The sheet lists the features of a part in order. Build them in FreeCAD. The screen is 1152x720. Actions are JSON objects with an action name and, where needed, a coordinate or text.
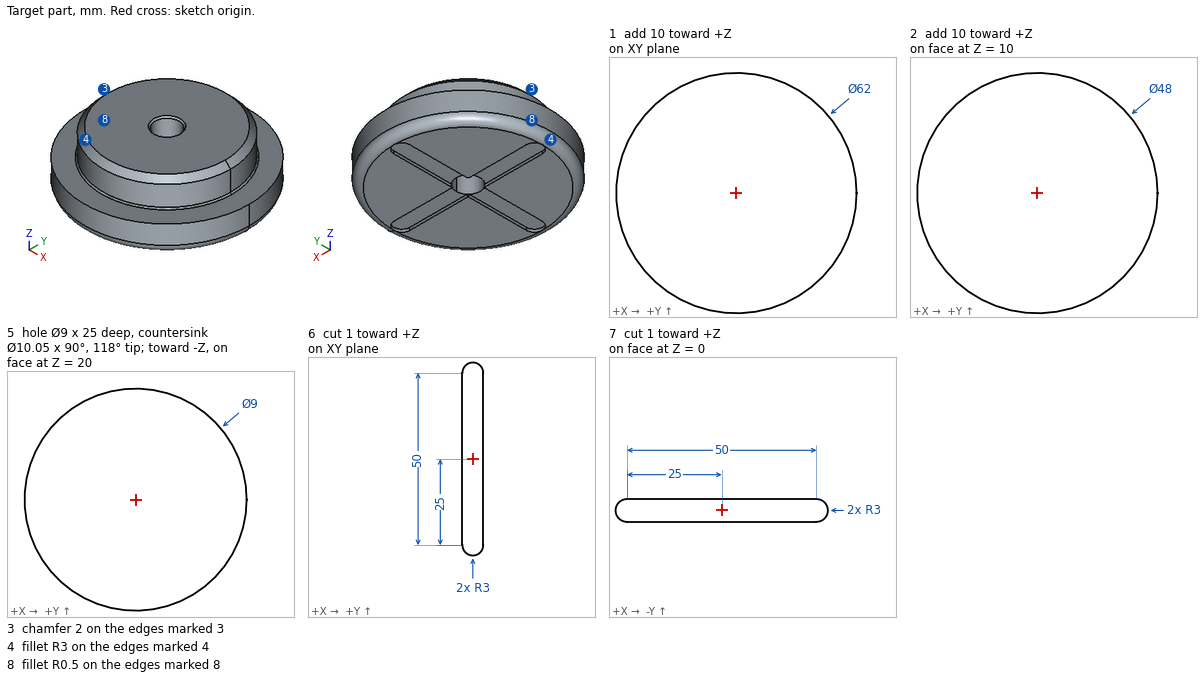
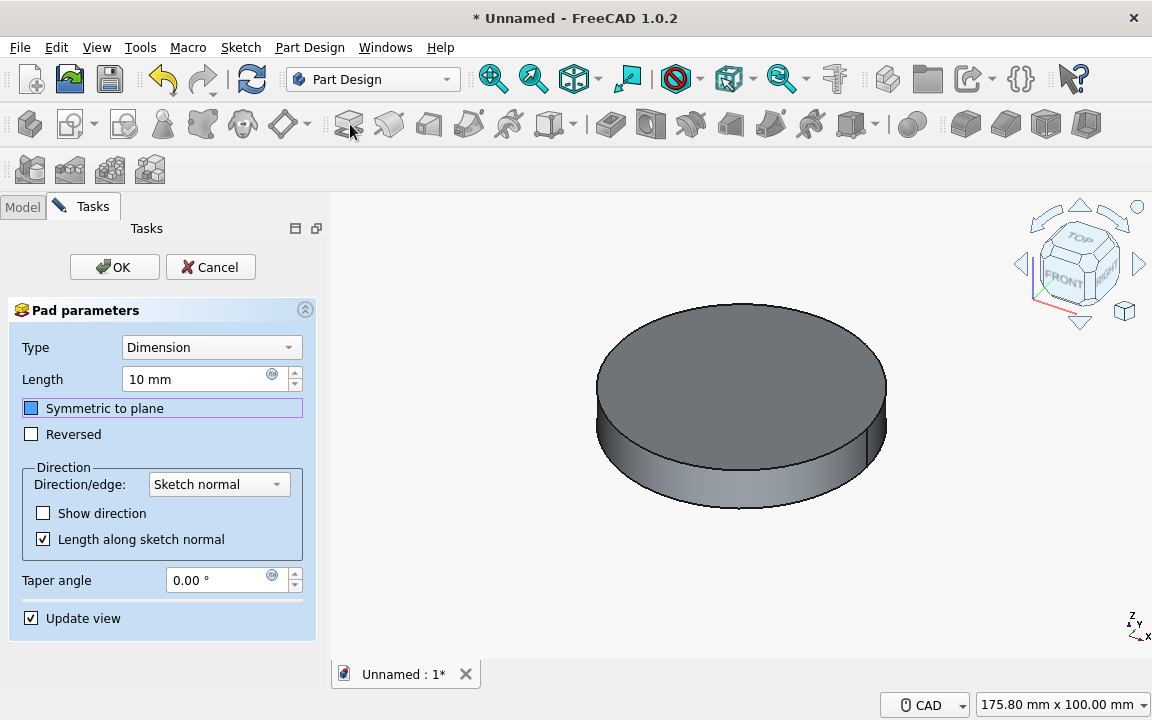
{"action": "left_click", "coordinate": [115, 267]}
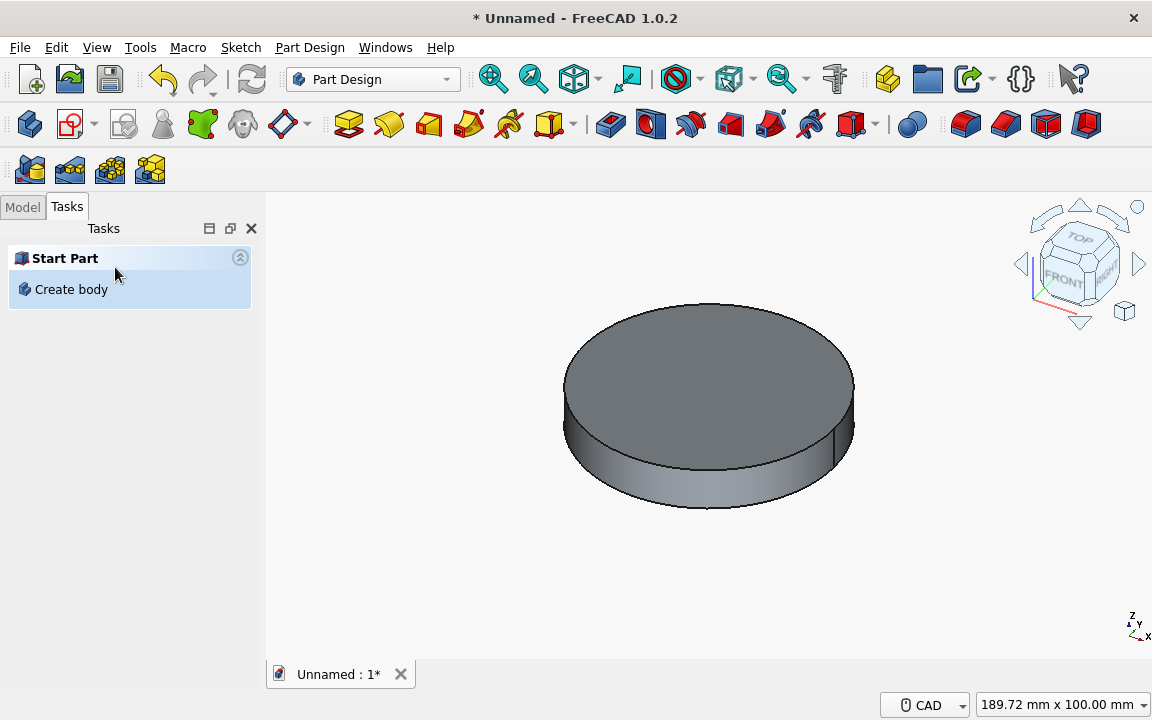
{"action": "left_click", "coordinate": [709, 386]}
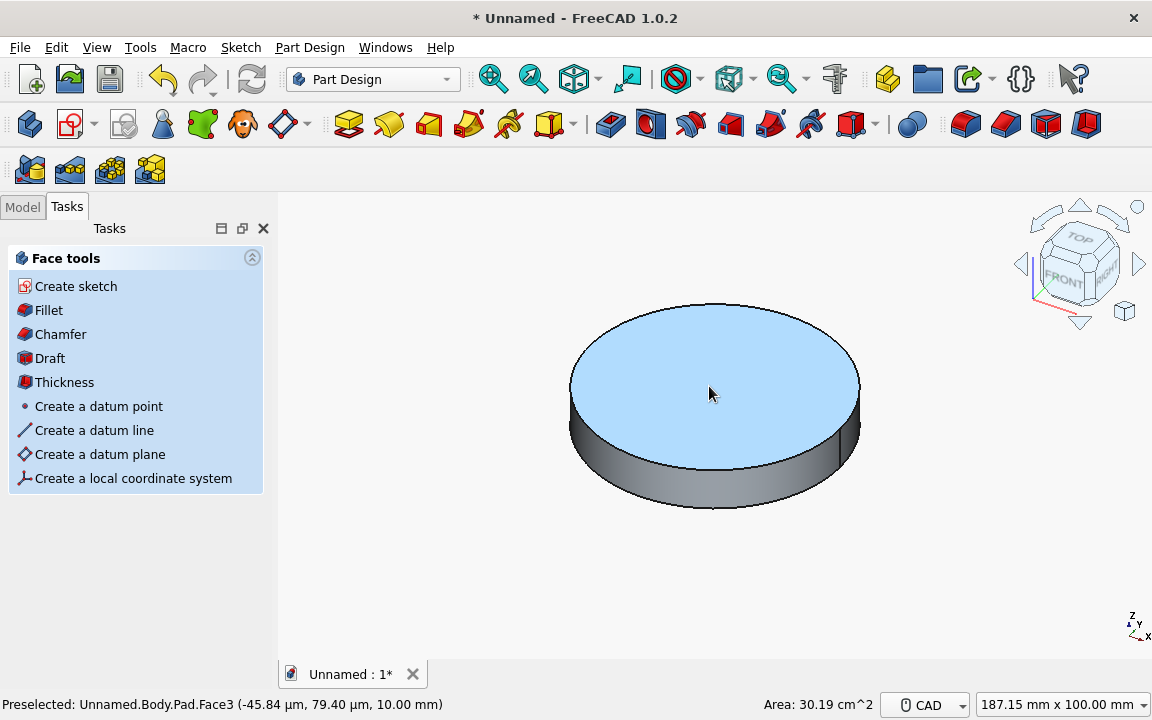
{"action": "left_click", "coordinate": [70, 124]}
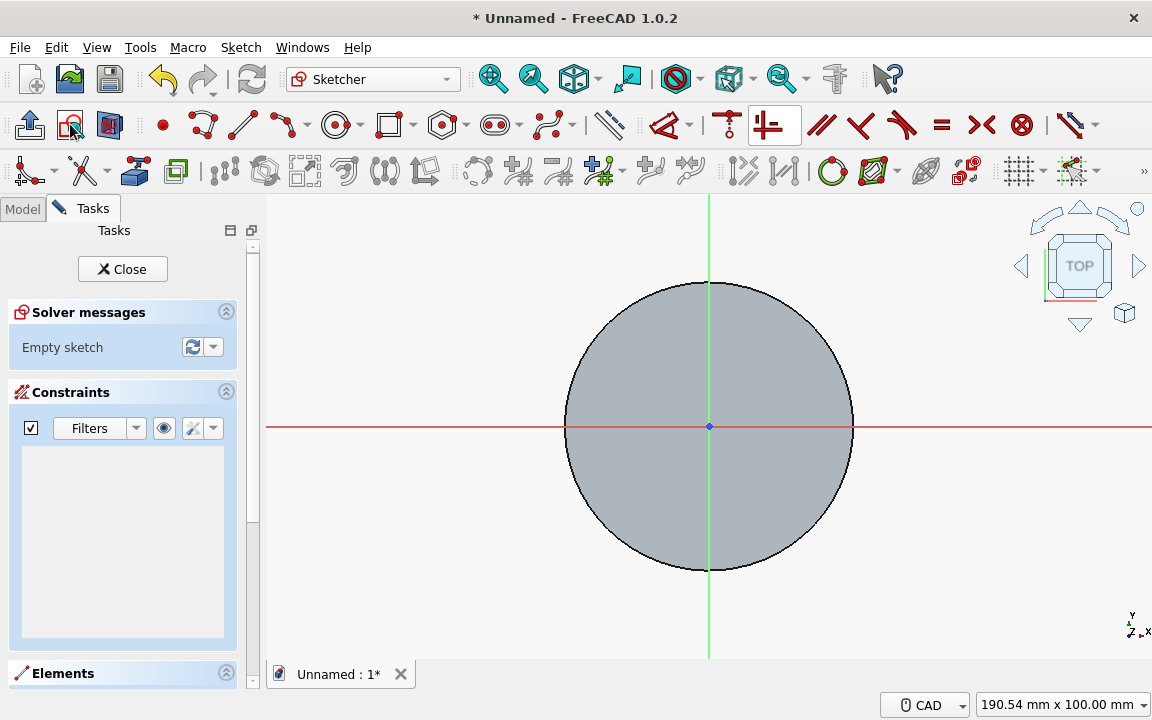
{"action": "key", "text": "g c"}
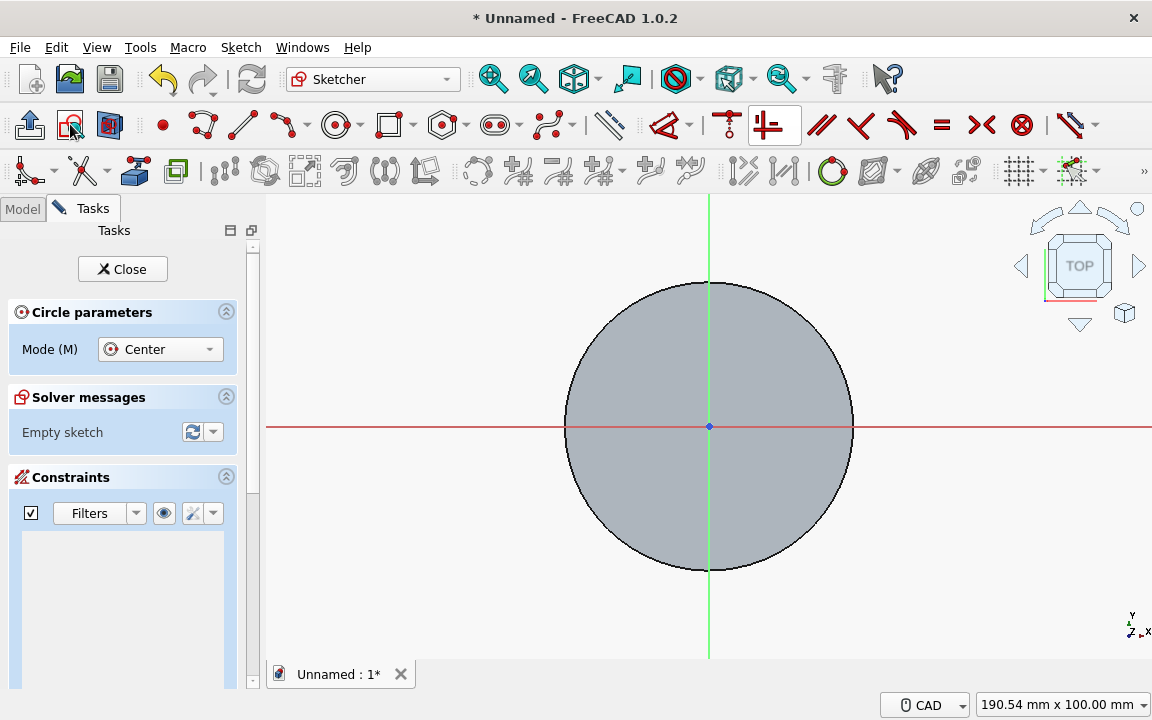
{"action": "left_click", "coordinate": [709, 426]}
{"action": "left_click", "coordinate": [788, 348]}
{"action": "key", "text": "Escape"}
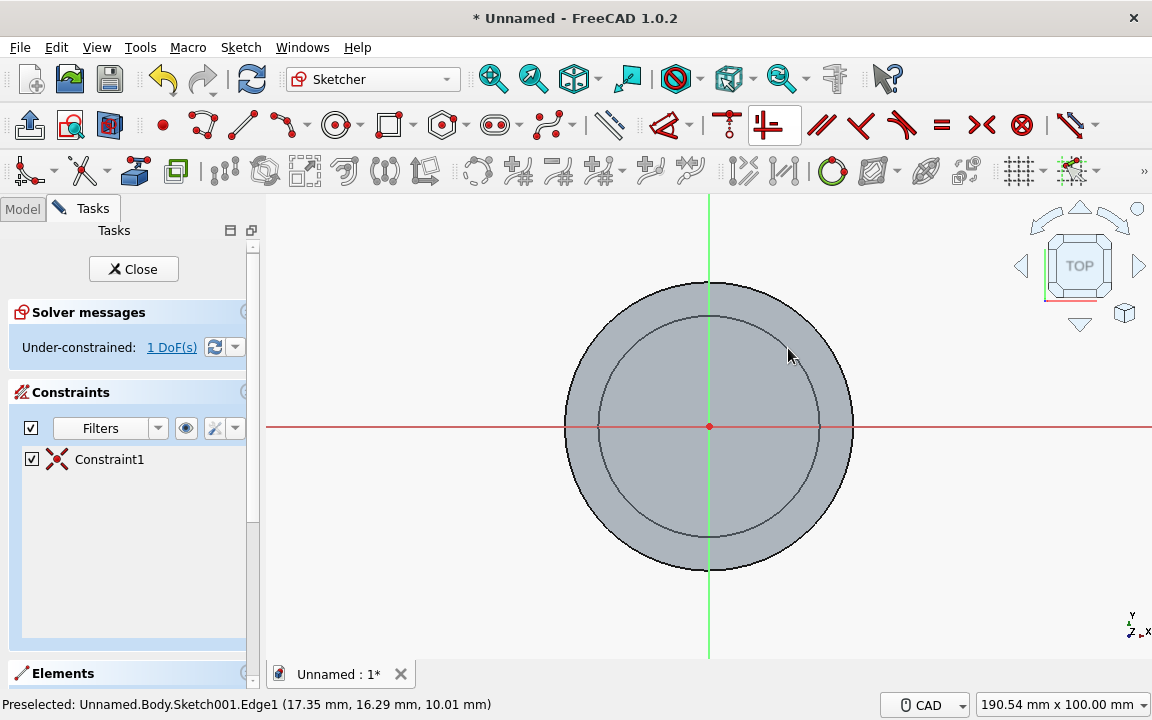
{"action": "left_click", "coordinate": [664, 126]}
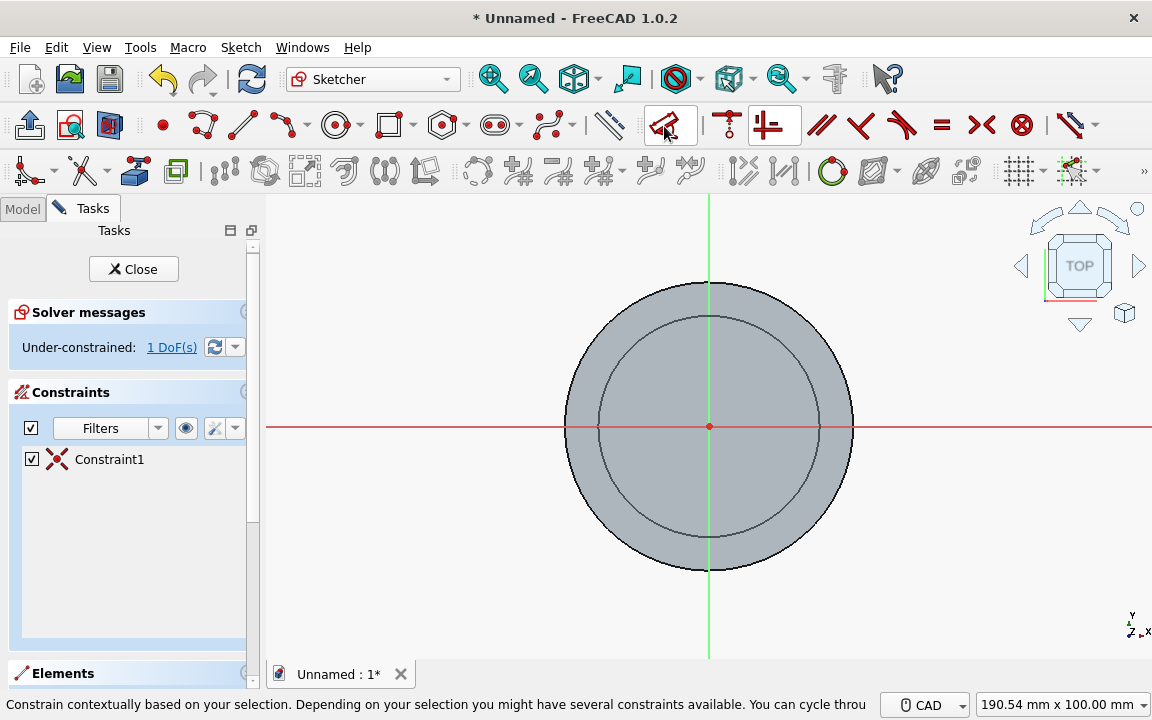
{"action": "left_click", "coordinate": [787, 348]}
{"action": "left_click", "coordinate": [810, 325]}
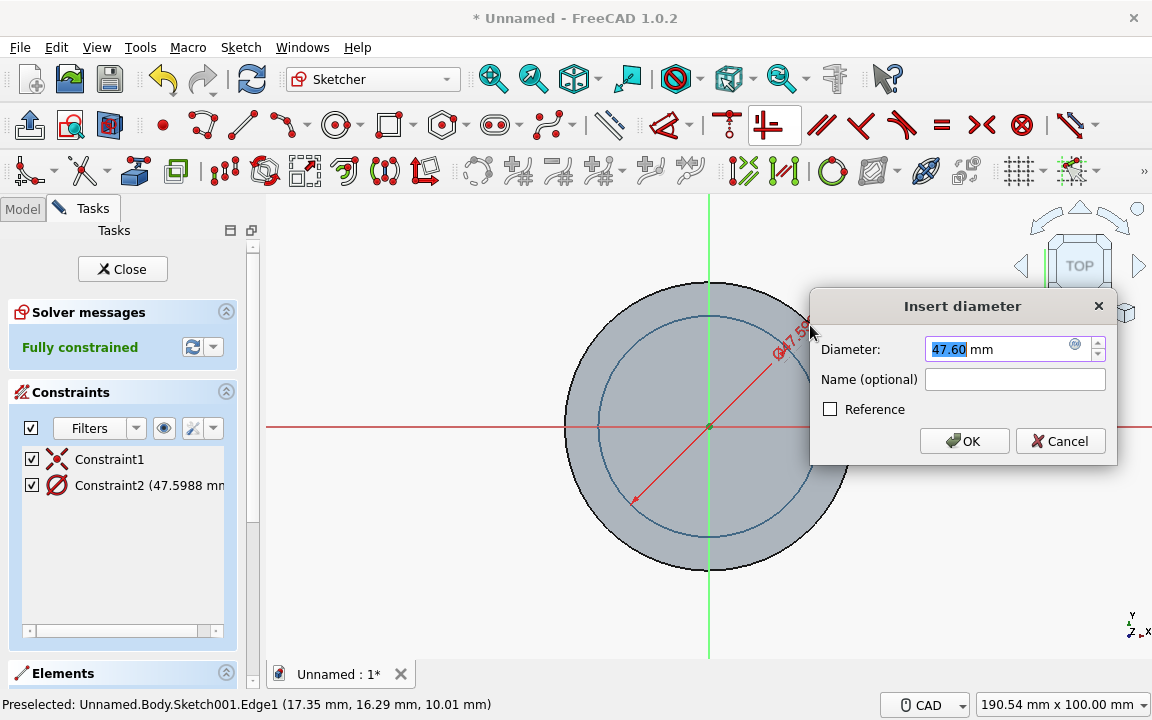
{"action": "type", "text": "48"}
{"action": "key", "text": "Return"}
{"action": "key", "text": "Escape"}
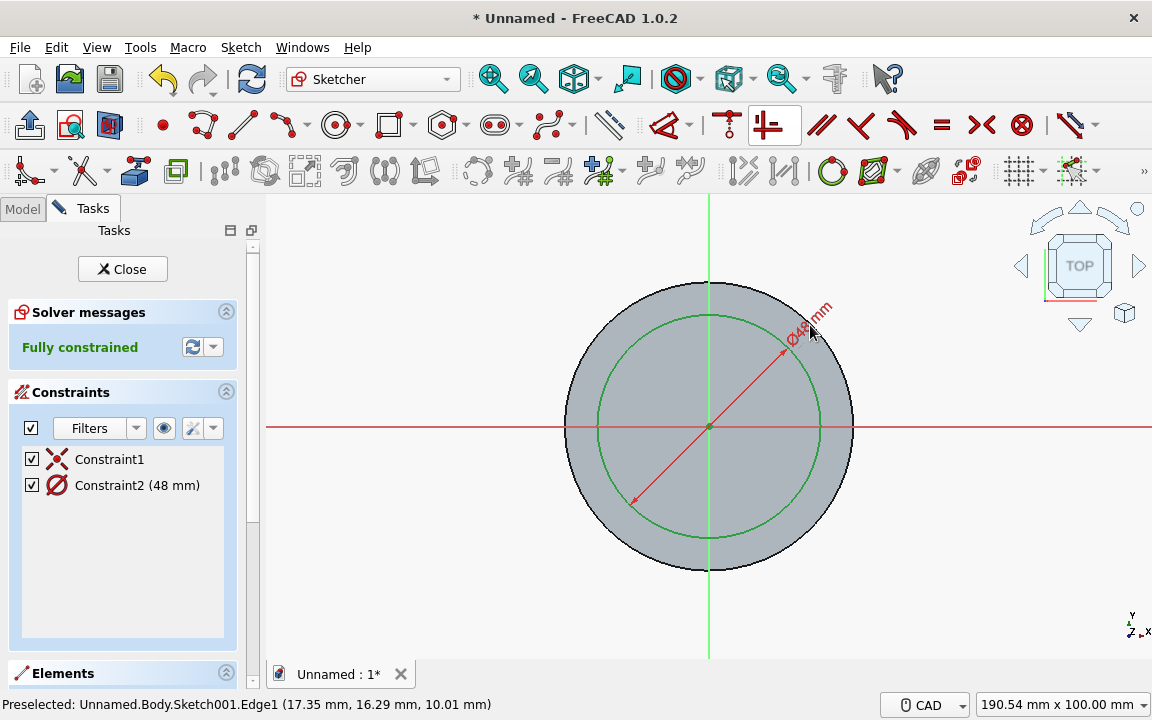
{"action": "left_click", "coordinate": [123, 269]}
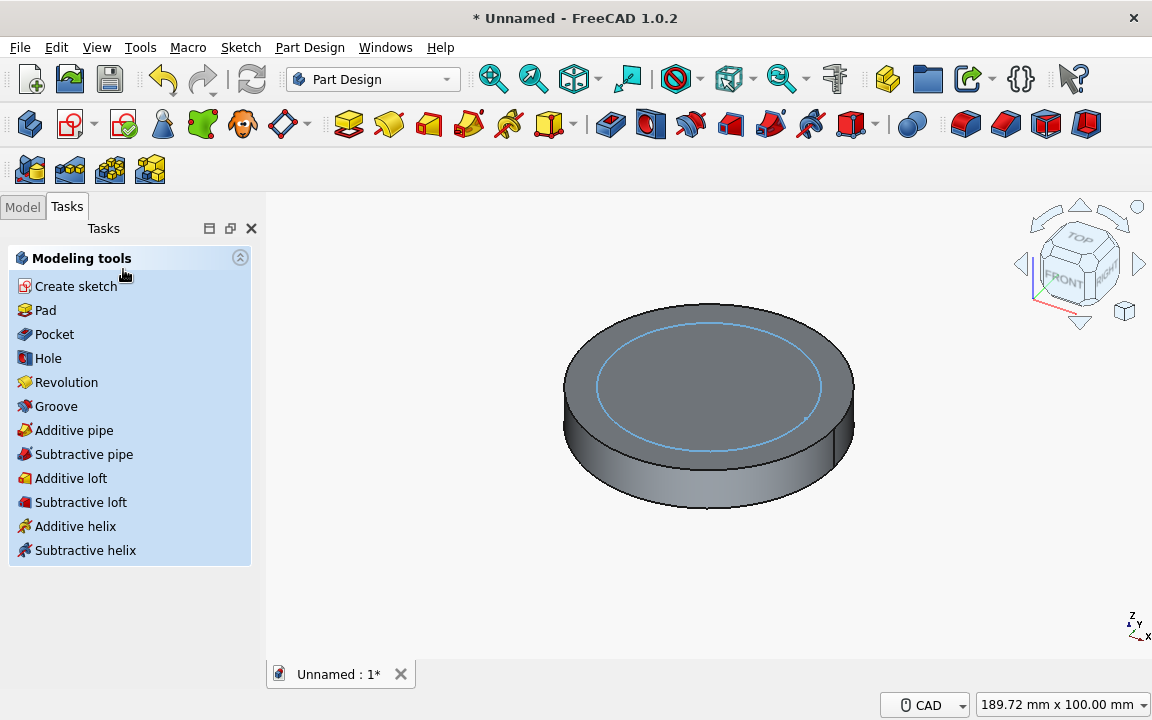
{"action": "left_click", "coordinate": [350, 124]}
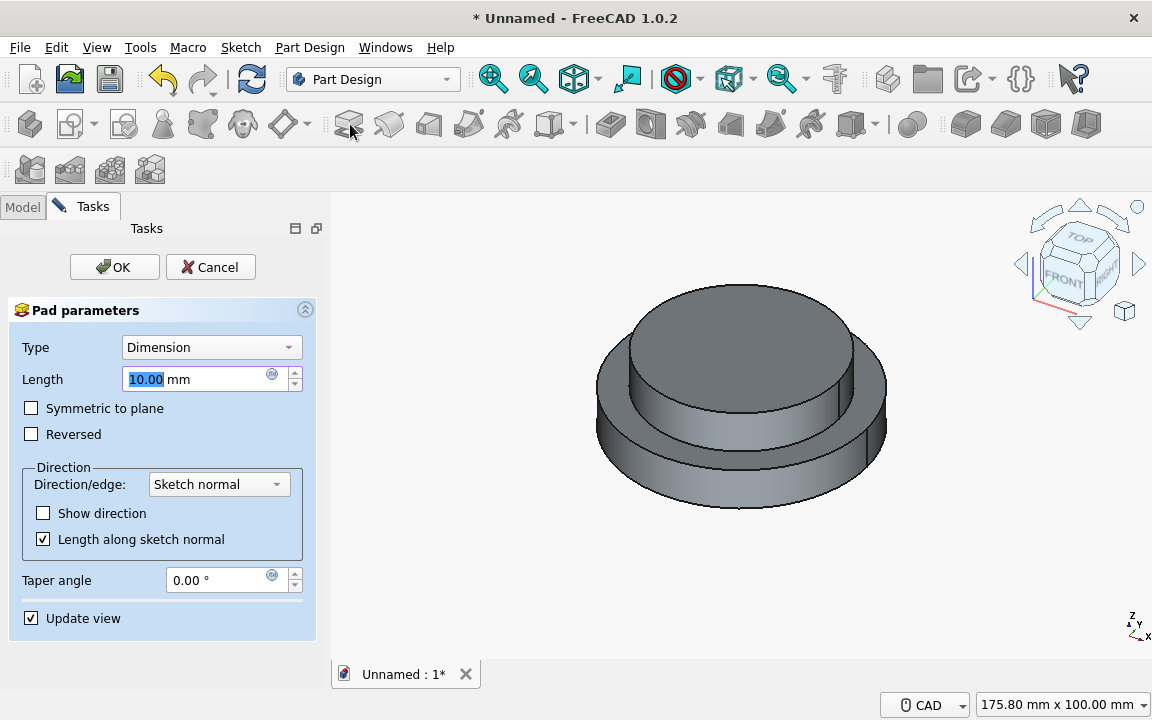
{"action": "type", "text": "10"}
{"action": "key", "text": "Tab"}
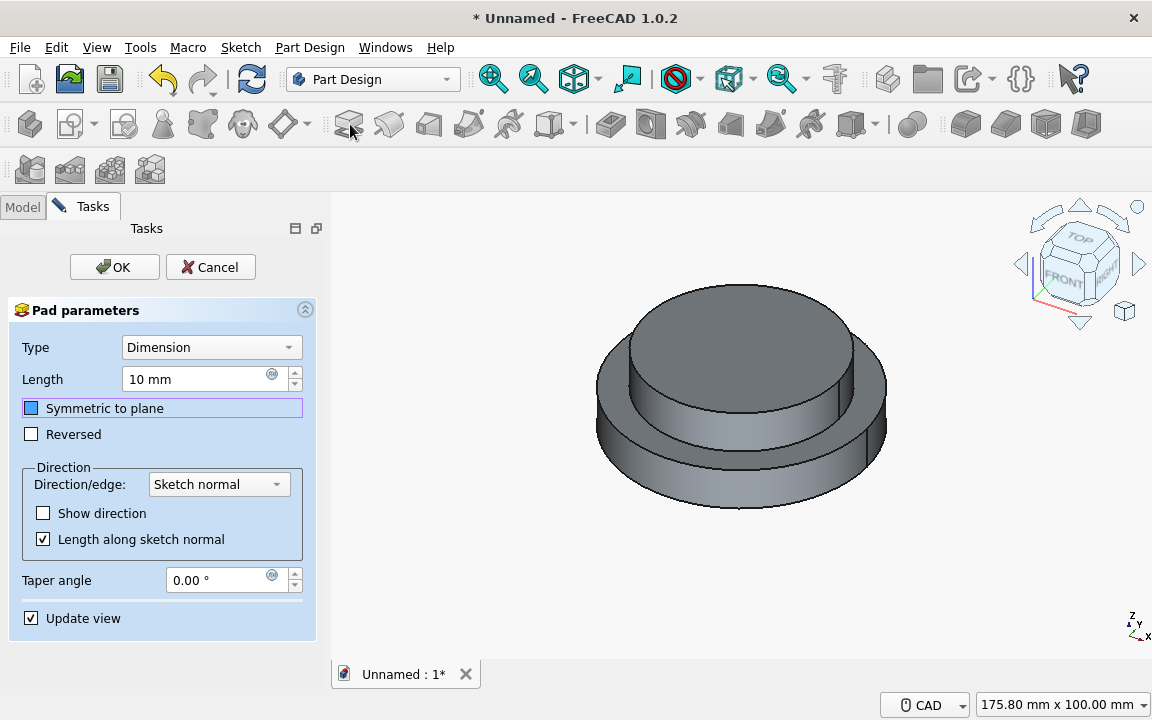
{"action": "left_click", "coordinate": [115, 267]}